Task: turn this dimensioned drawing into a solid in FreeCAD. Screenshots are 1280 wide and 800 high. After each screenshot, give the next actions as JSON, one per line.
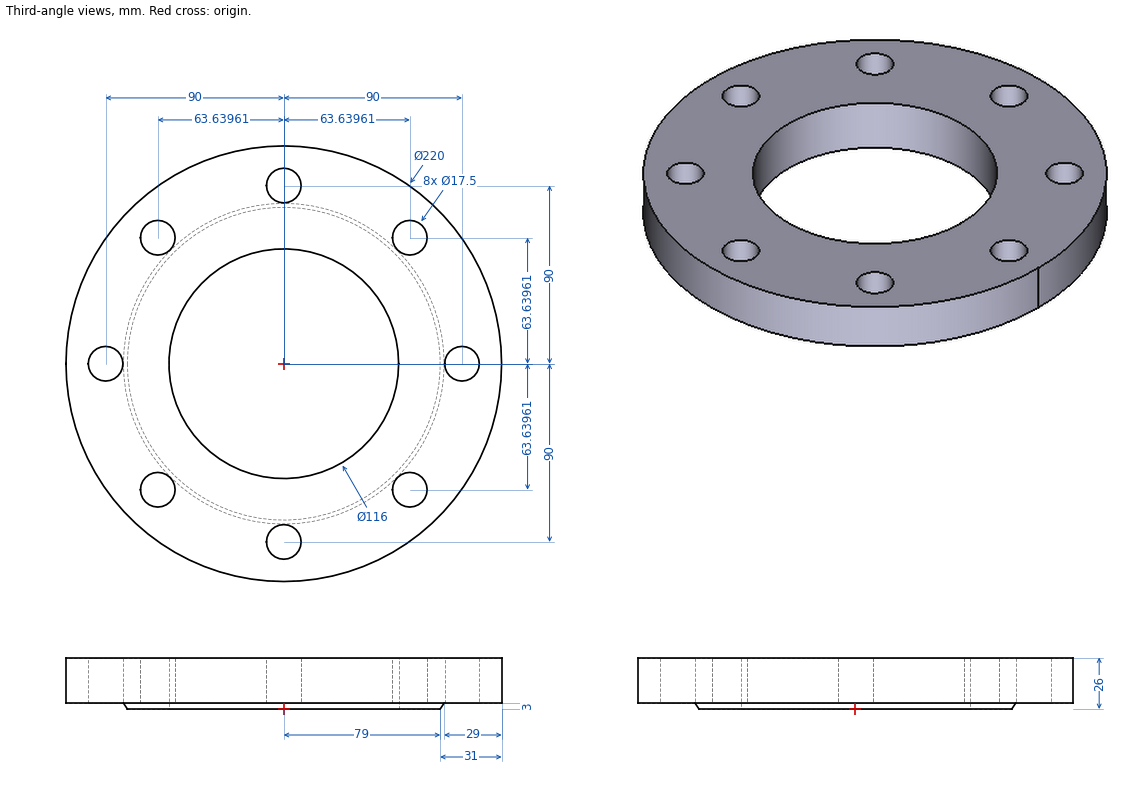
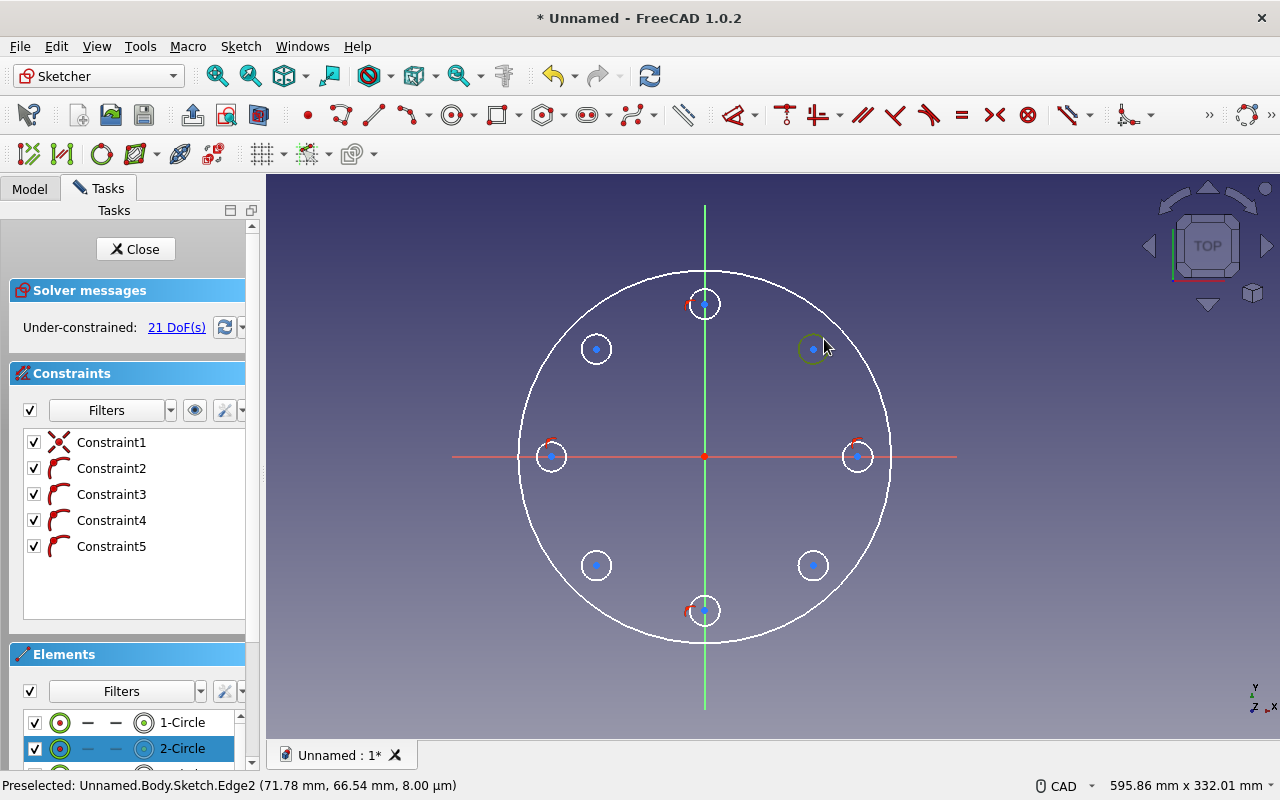
{"action": "scroll", "coordinate": [715, 294], "scroll_direction": "up", "scroll_amount": 2}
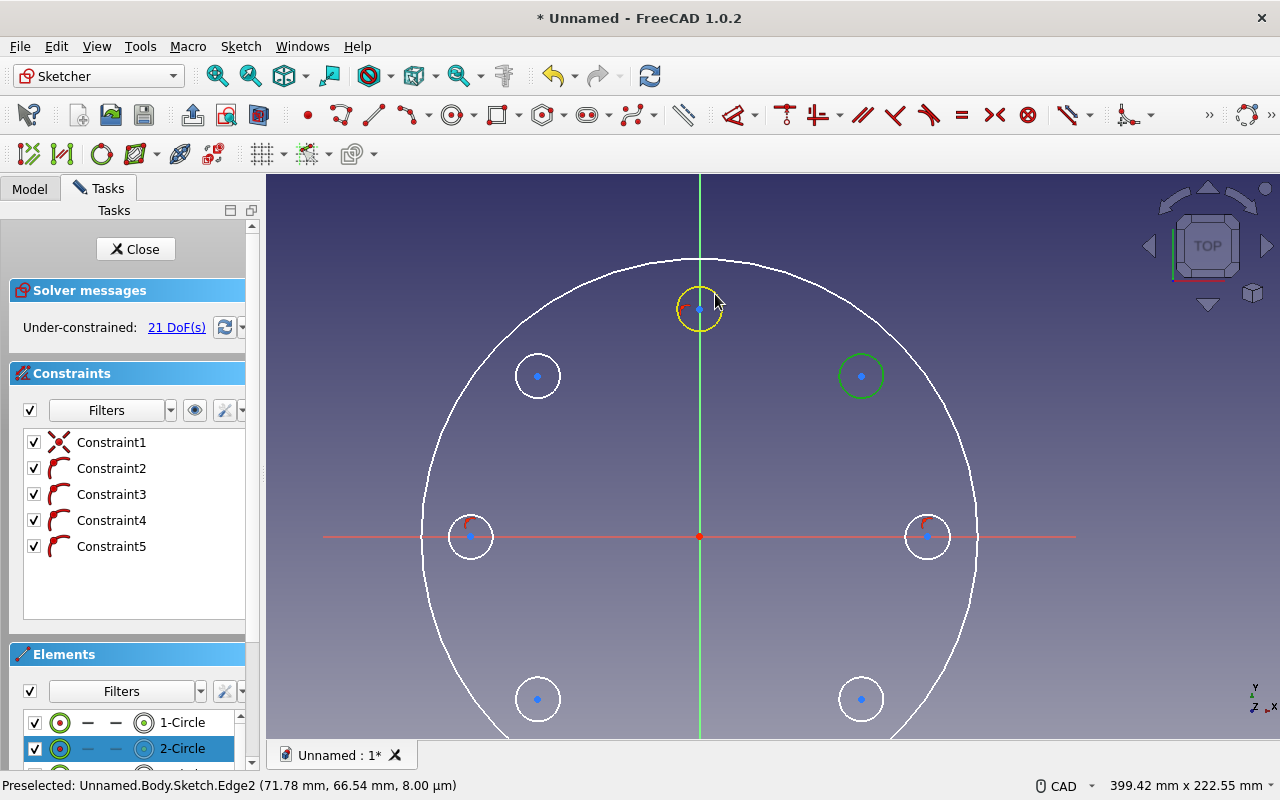
{"action": "left_click", "coordinate": [715, 293]}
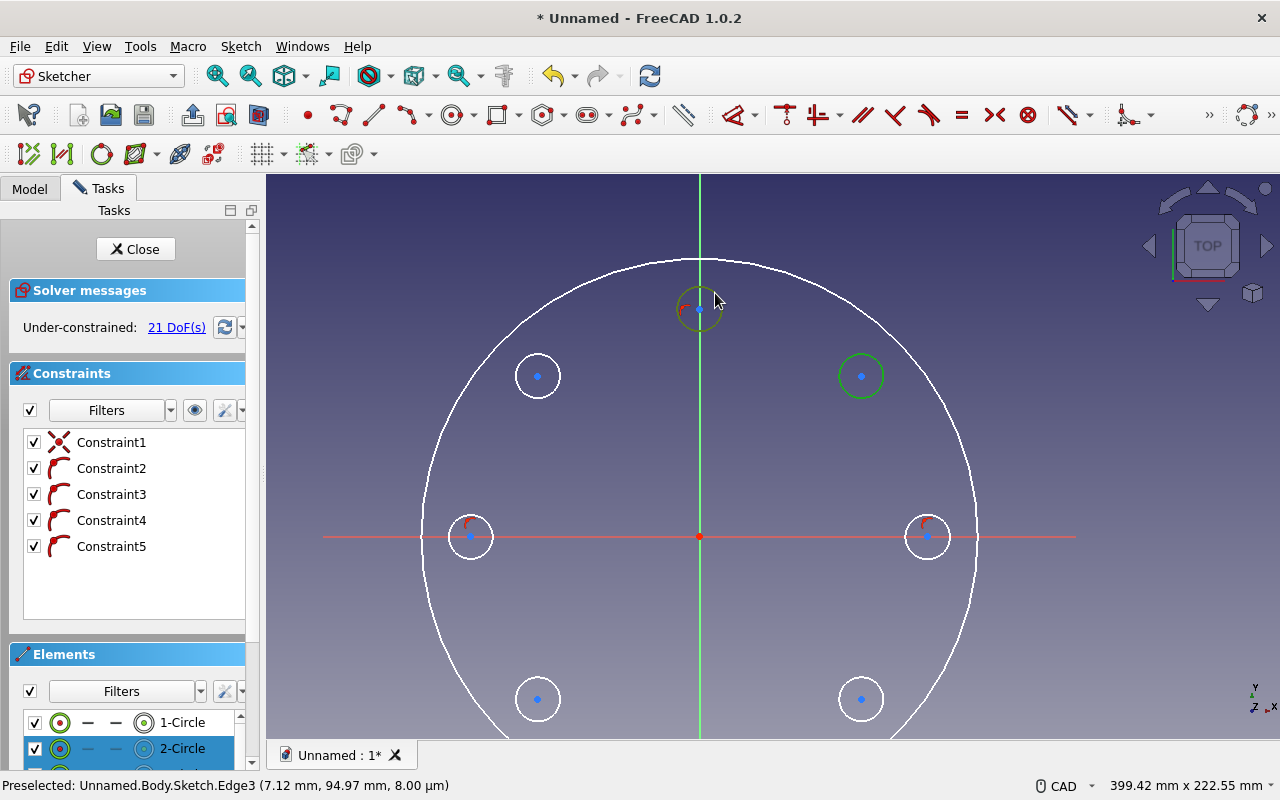
{"action": "left_click", "coordinate": [553, 361]}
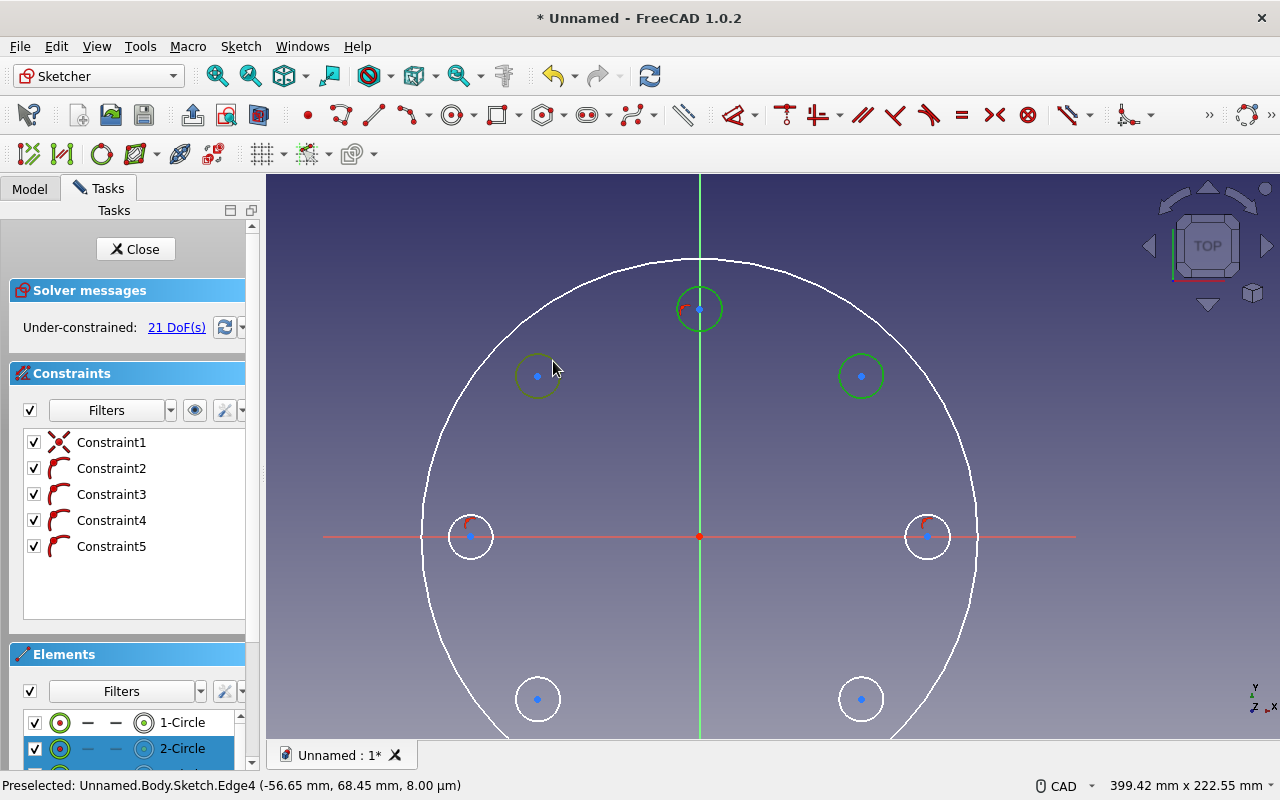
{"action": "left_click", "coordinate": [943, 521]}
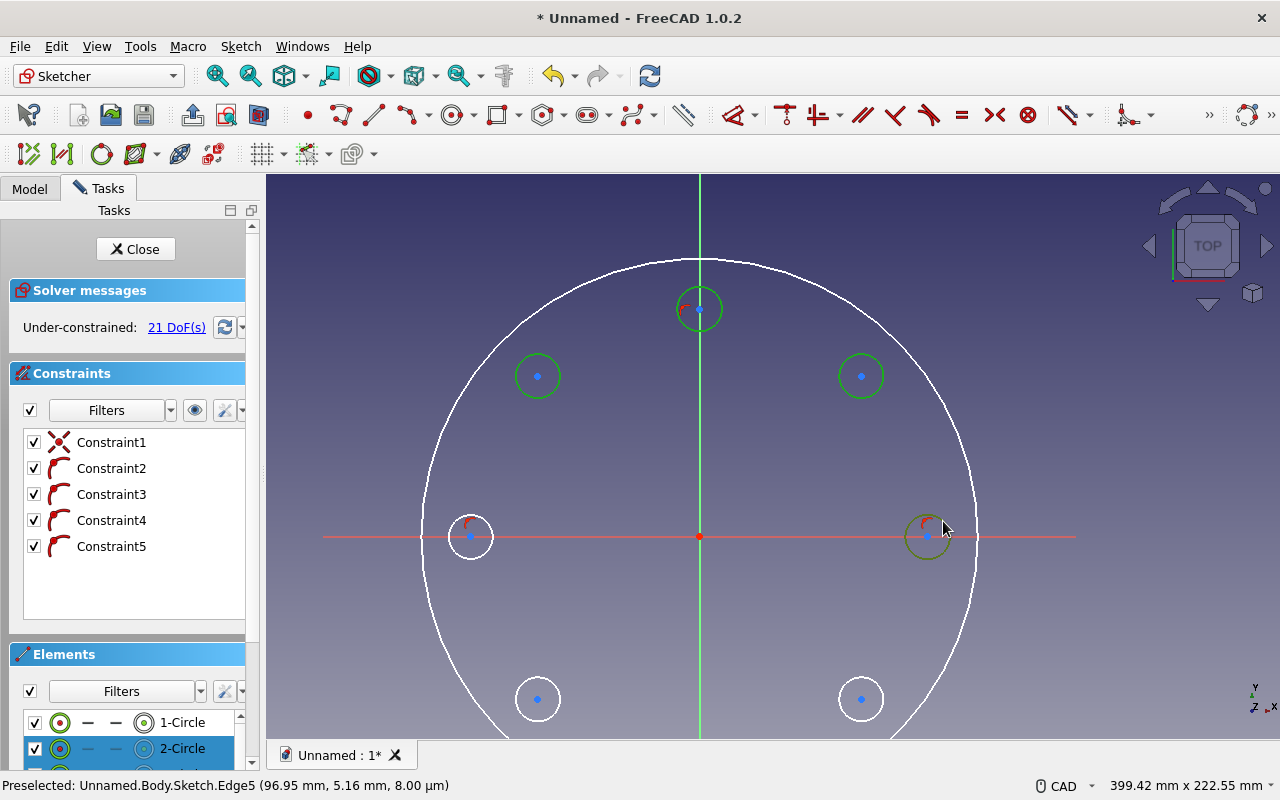
{"action": "left_click", "coordinate": [877, 684]}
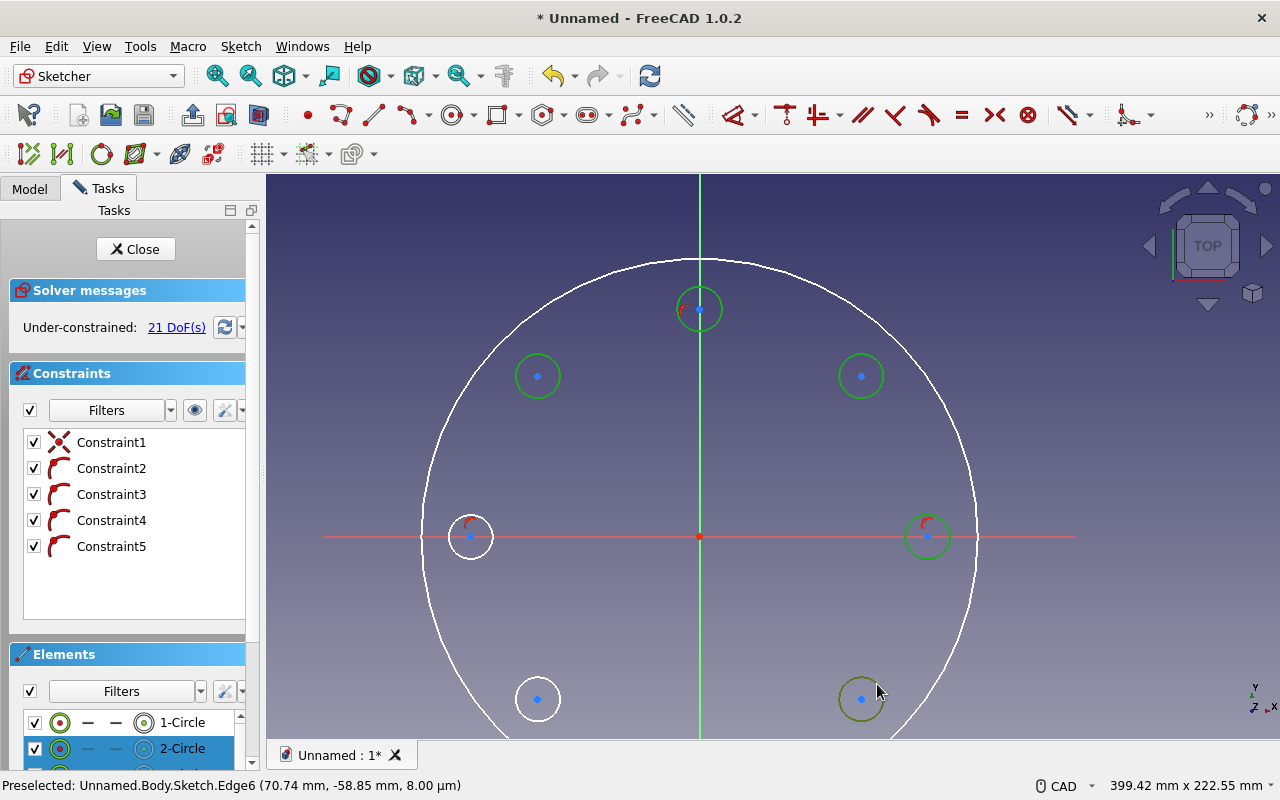
{"action": "left_click", "coordinate": [486, 521]}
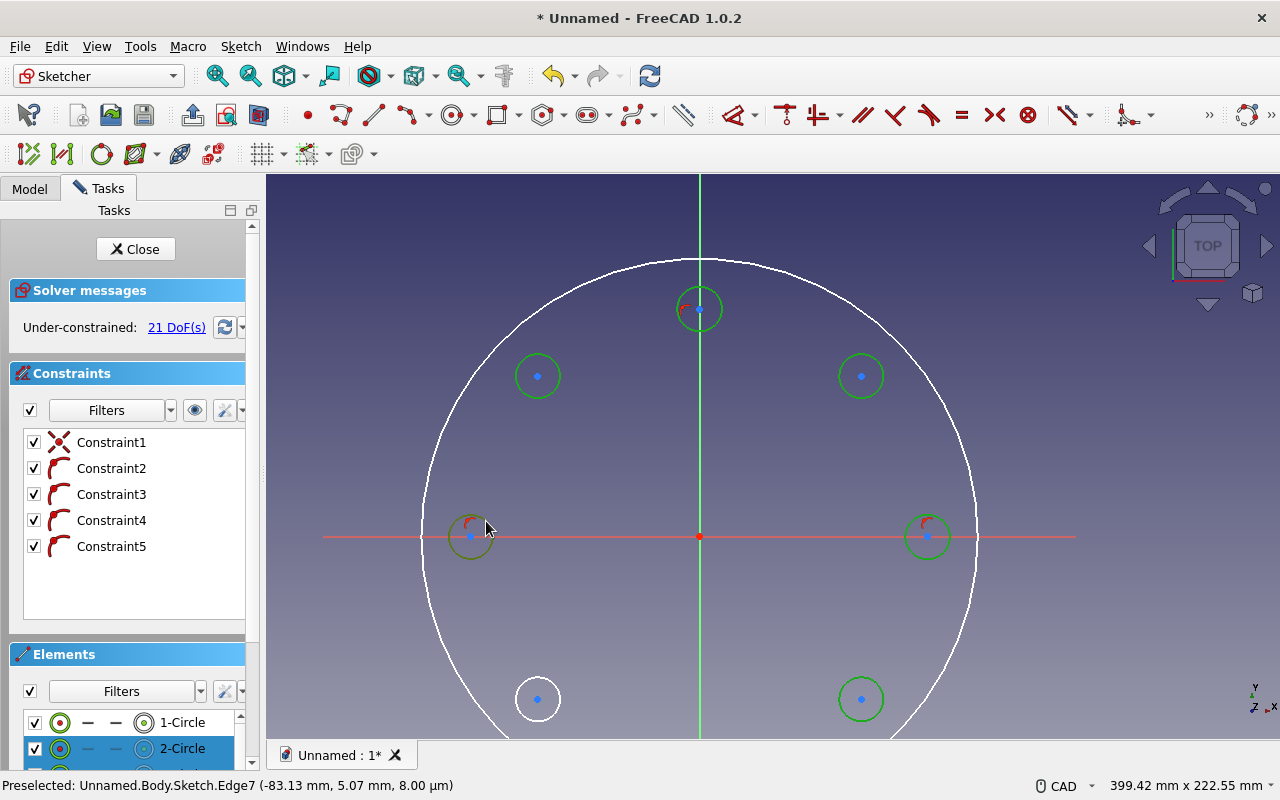
{"action": "scroll", "coordinate": [715, 293], "scroll_direction": "down", "scroll_amount": 2}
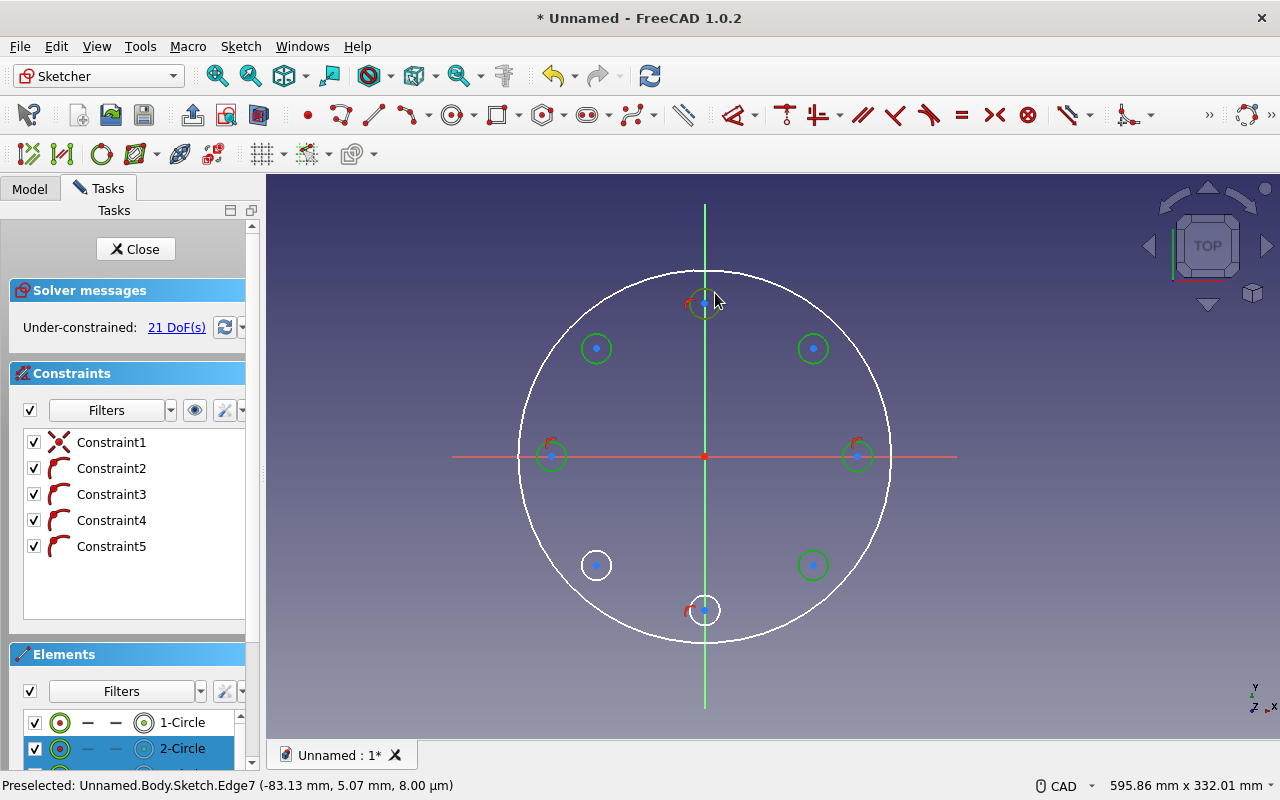
{"action": "scroll", "coordinate": [715, 600], "scroll_direction": "up", "scroll_amount": 2}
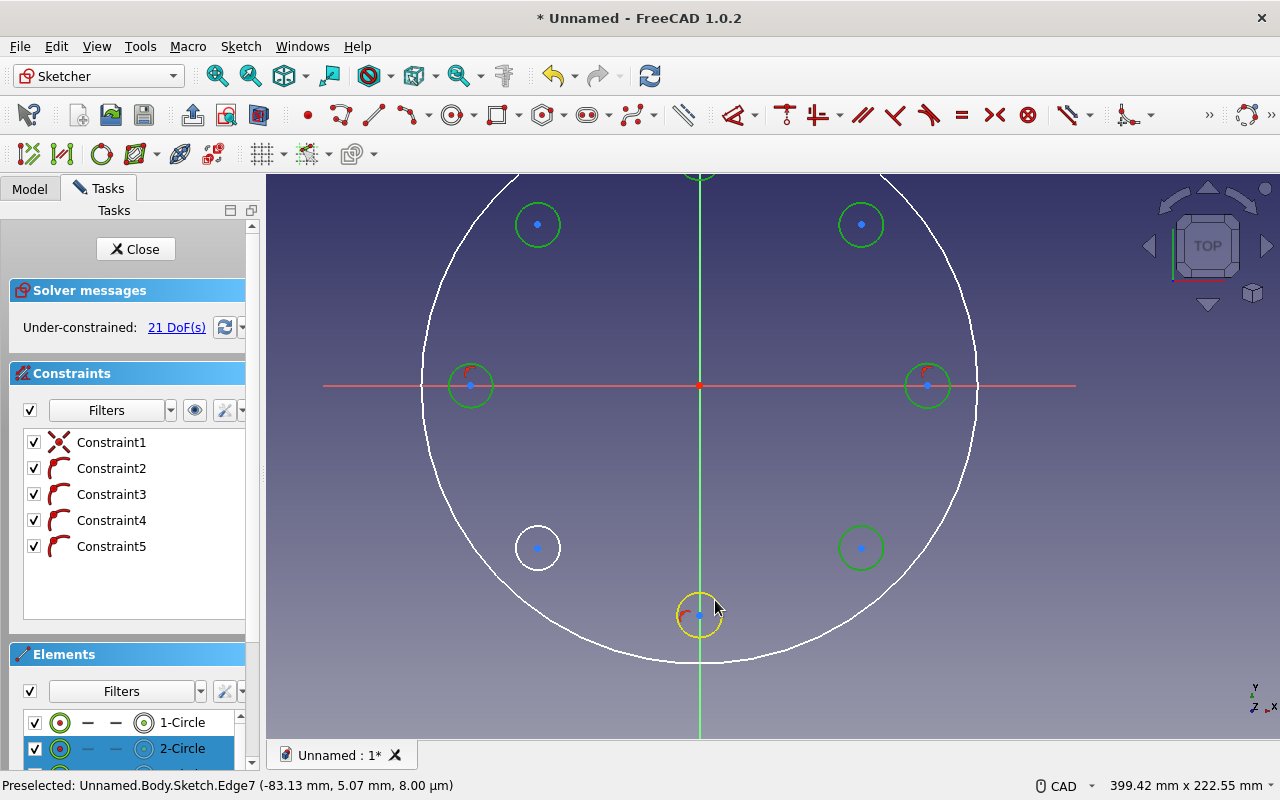
{"action": "left_click", "coordinate": [715, 599]}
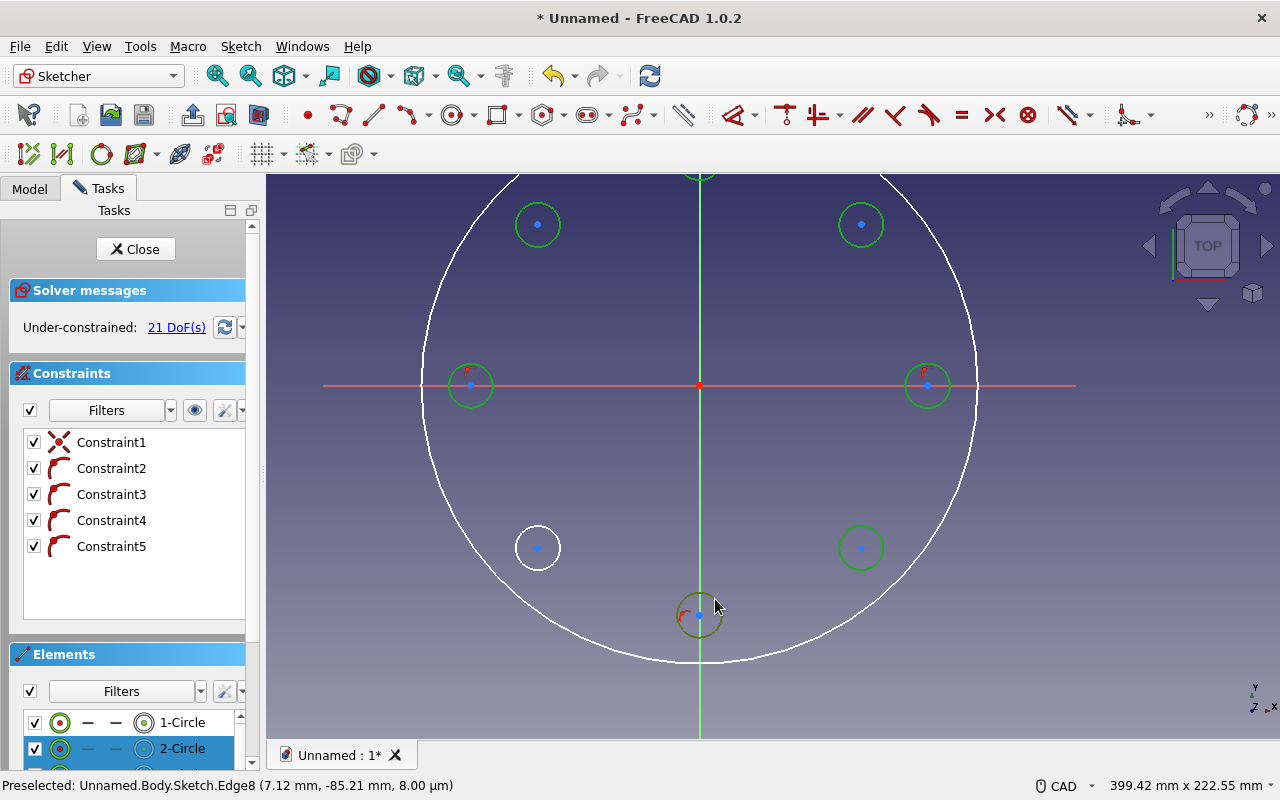
{"action": "left_click", "coordinate": [553, 532]}